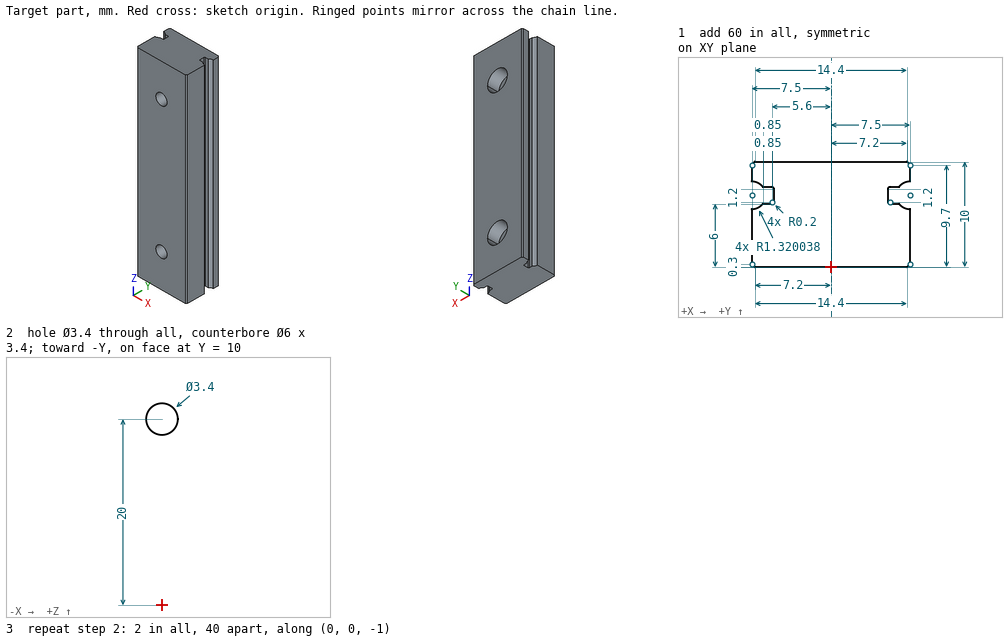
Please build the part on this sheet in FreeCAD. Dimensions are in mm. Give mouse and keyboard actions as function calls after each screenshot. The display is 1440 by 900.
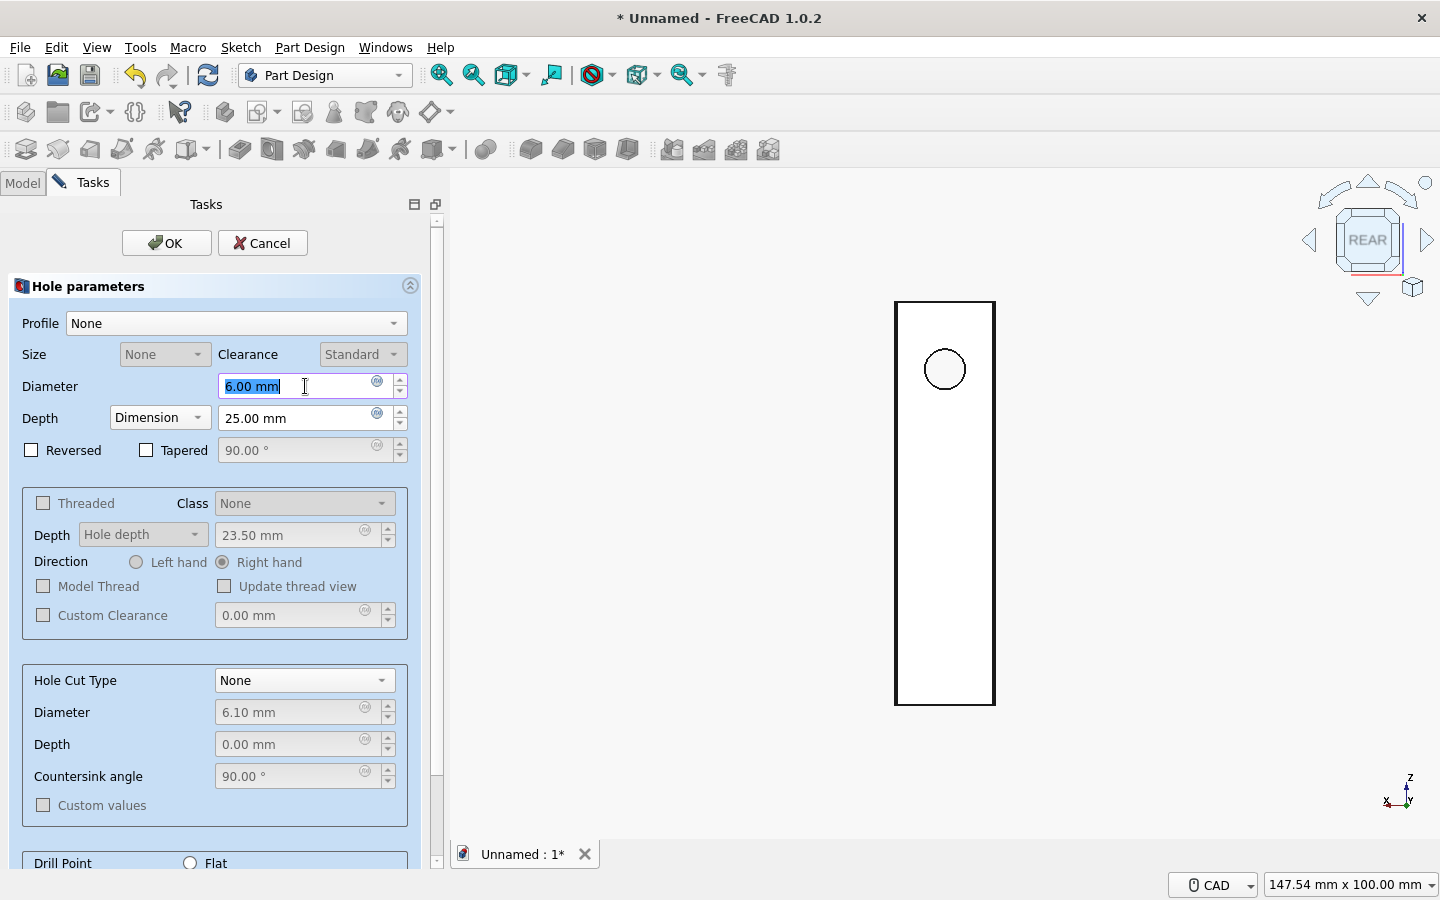
text(3.4)
key(Tab)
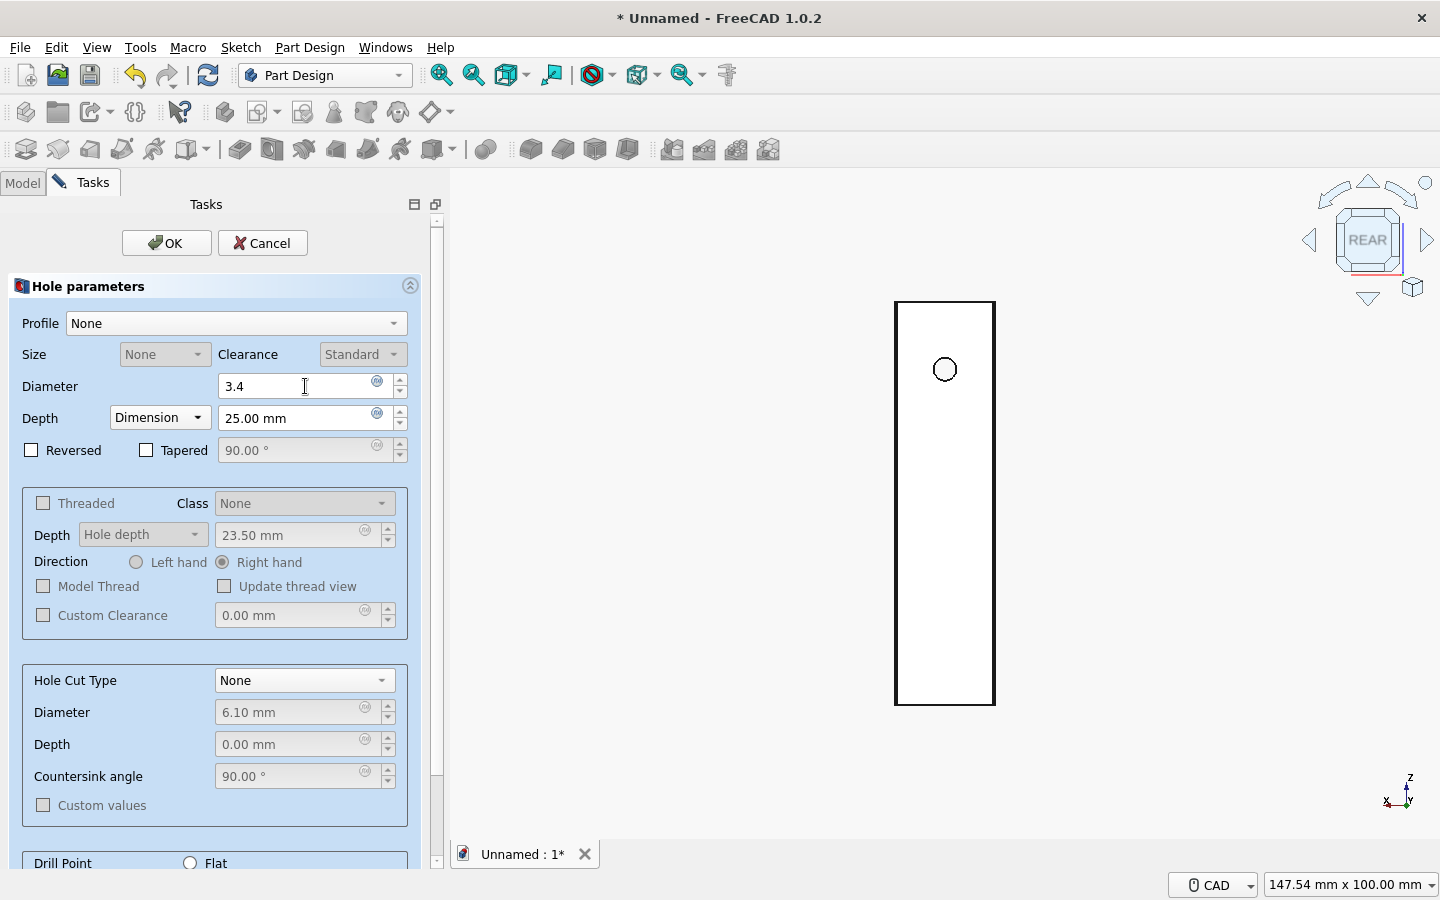
click(161, 418)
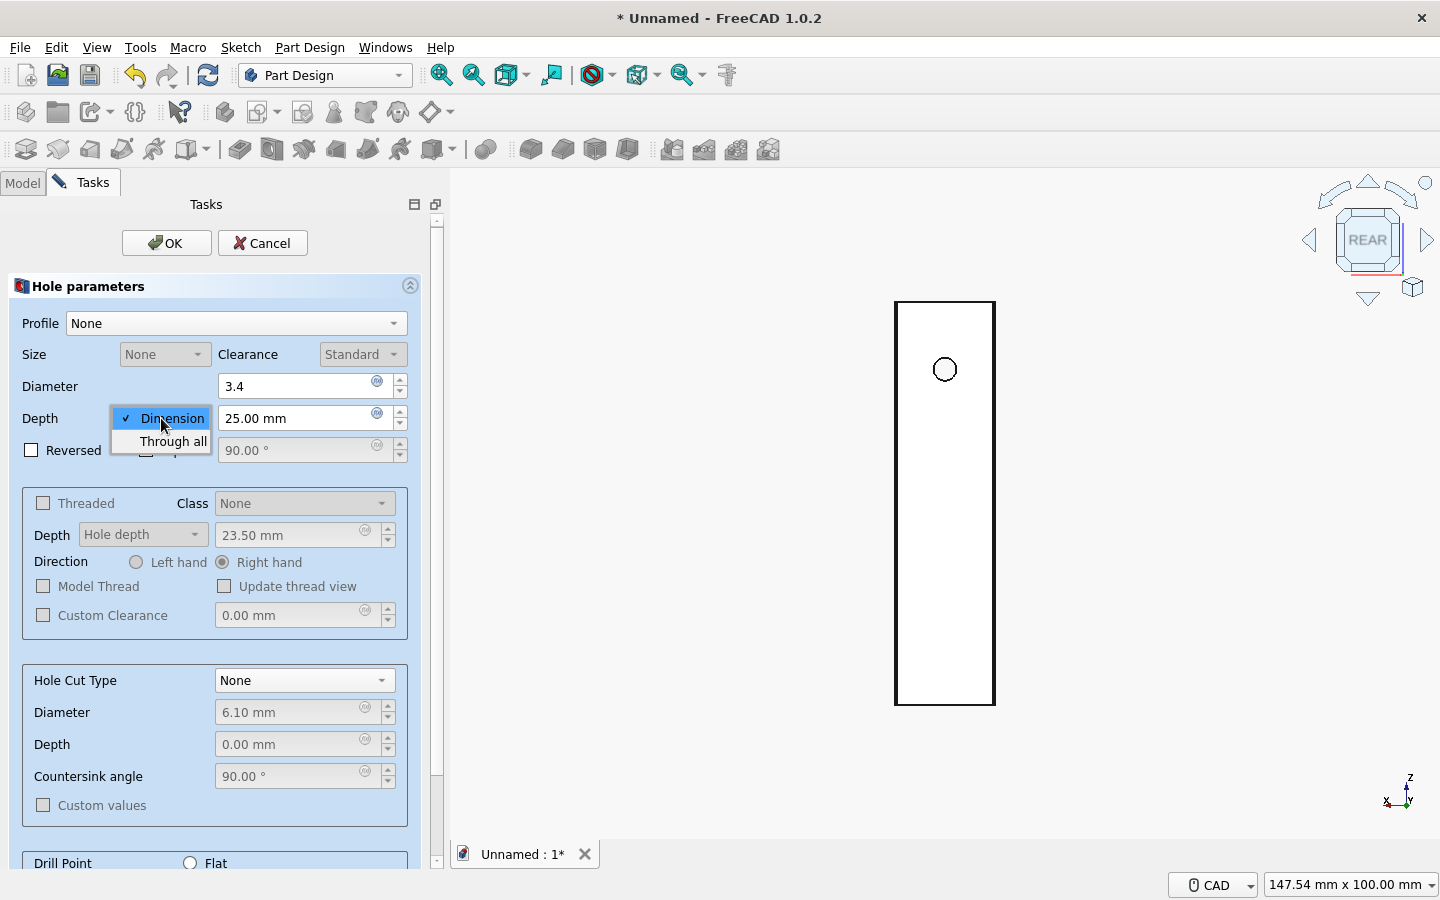
click(160, 442)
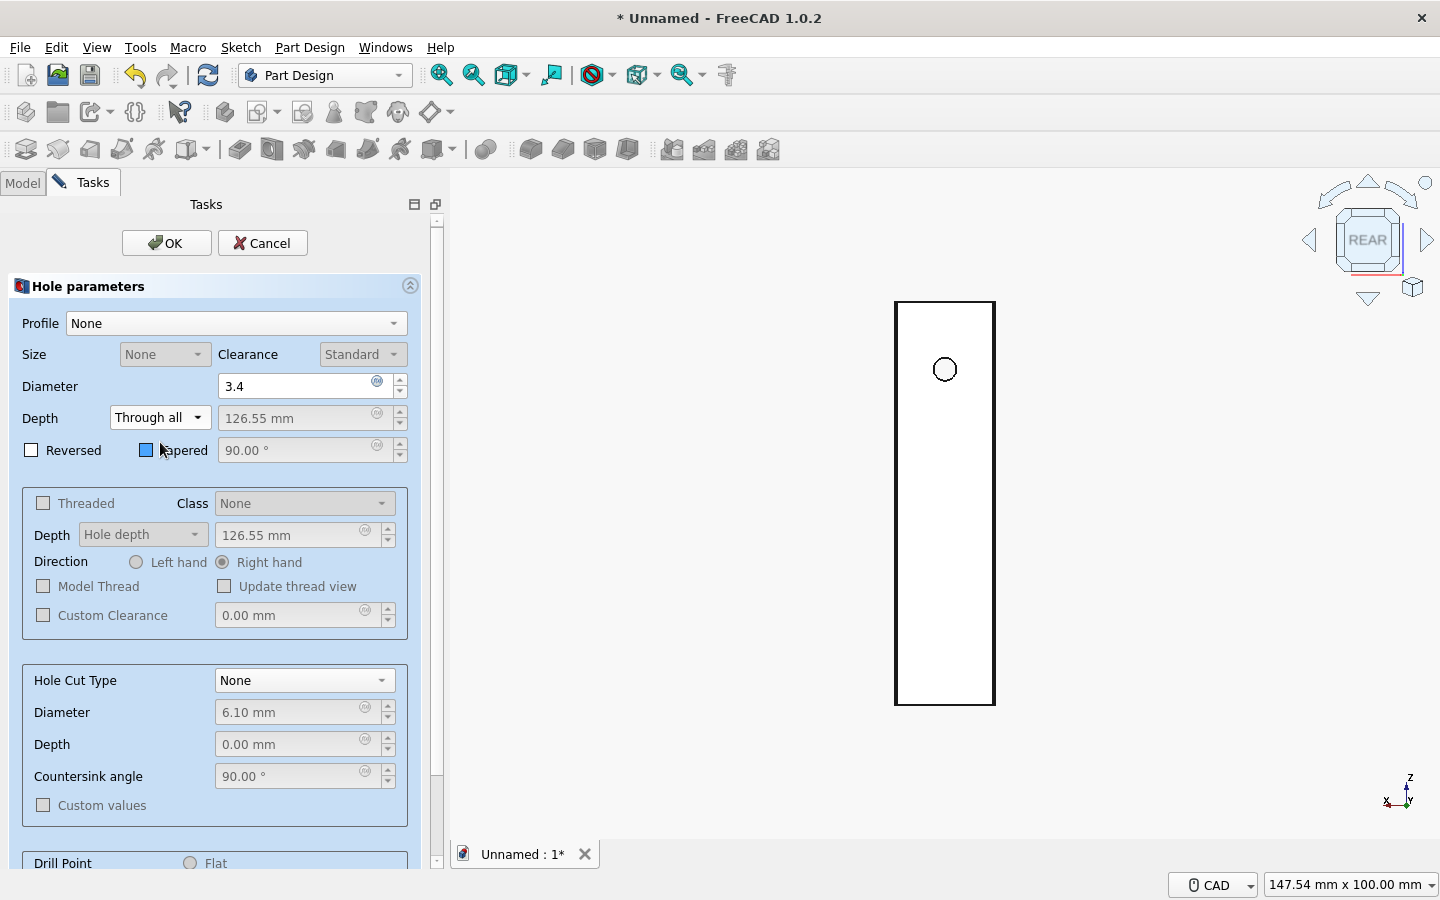
click(306, 680)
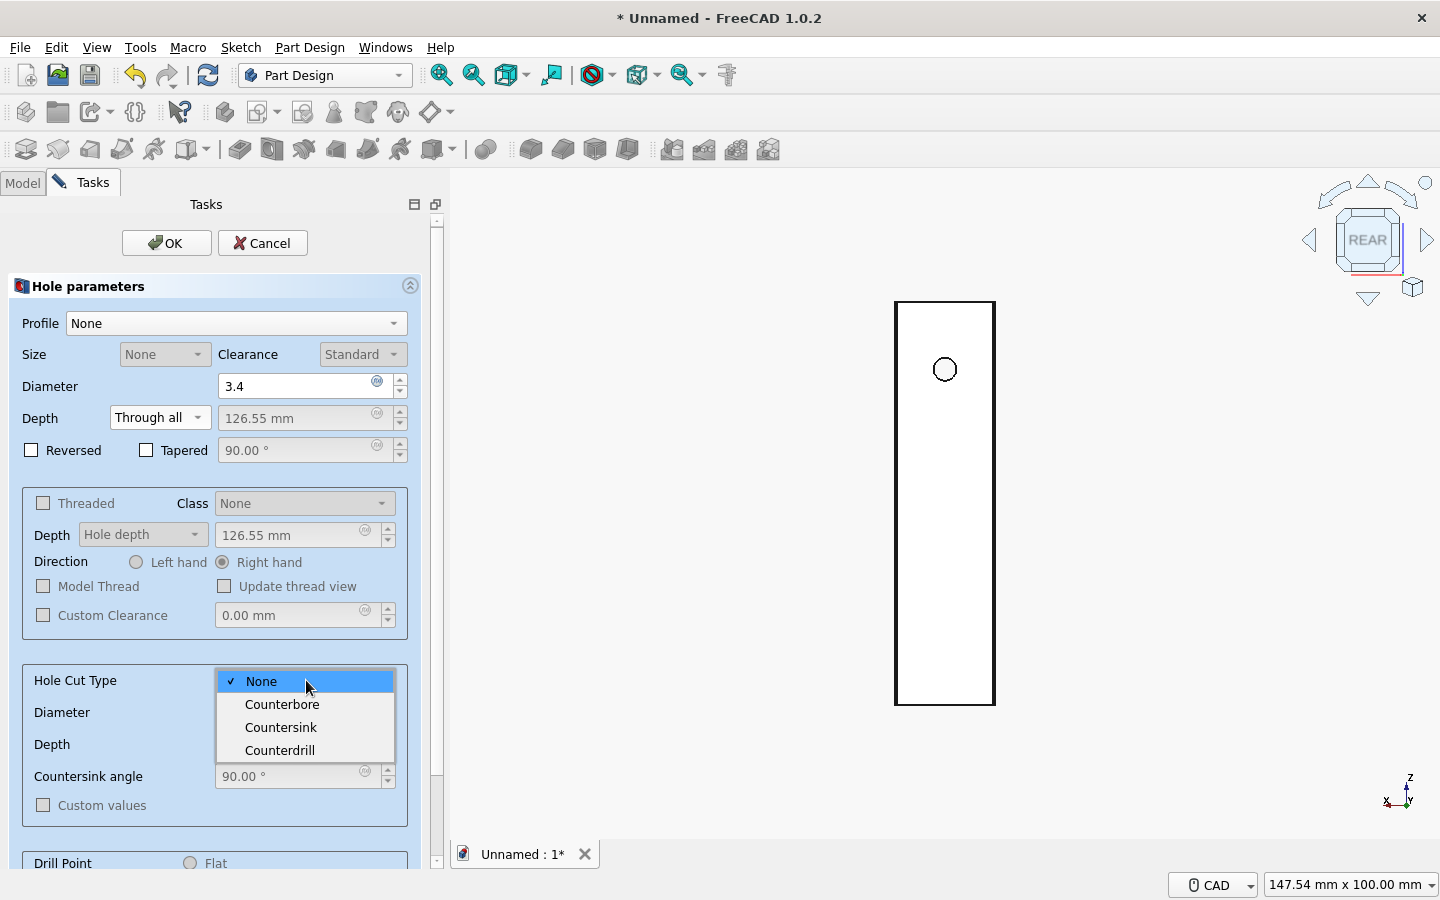
click(304, 704)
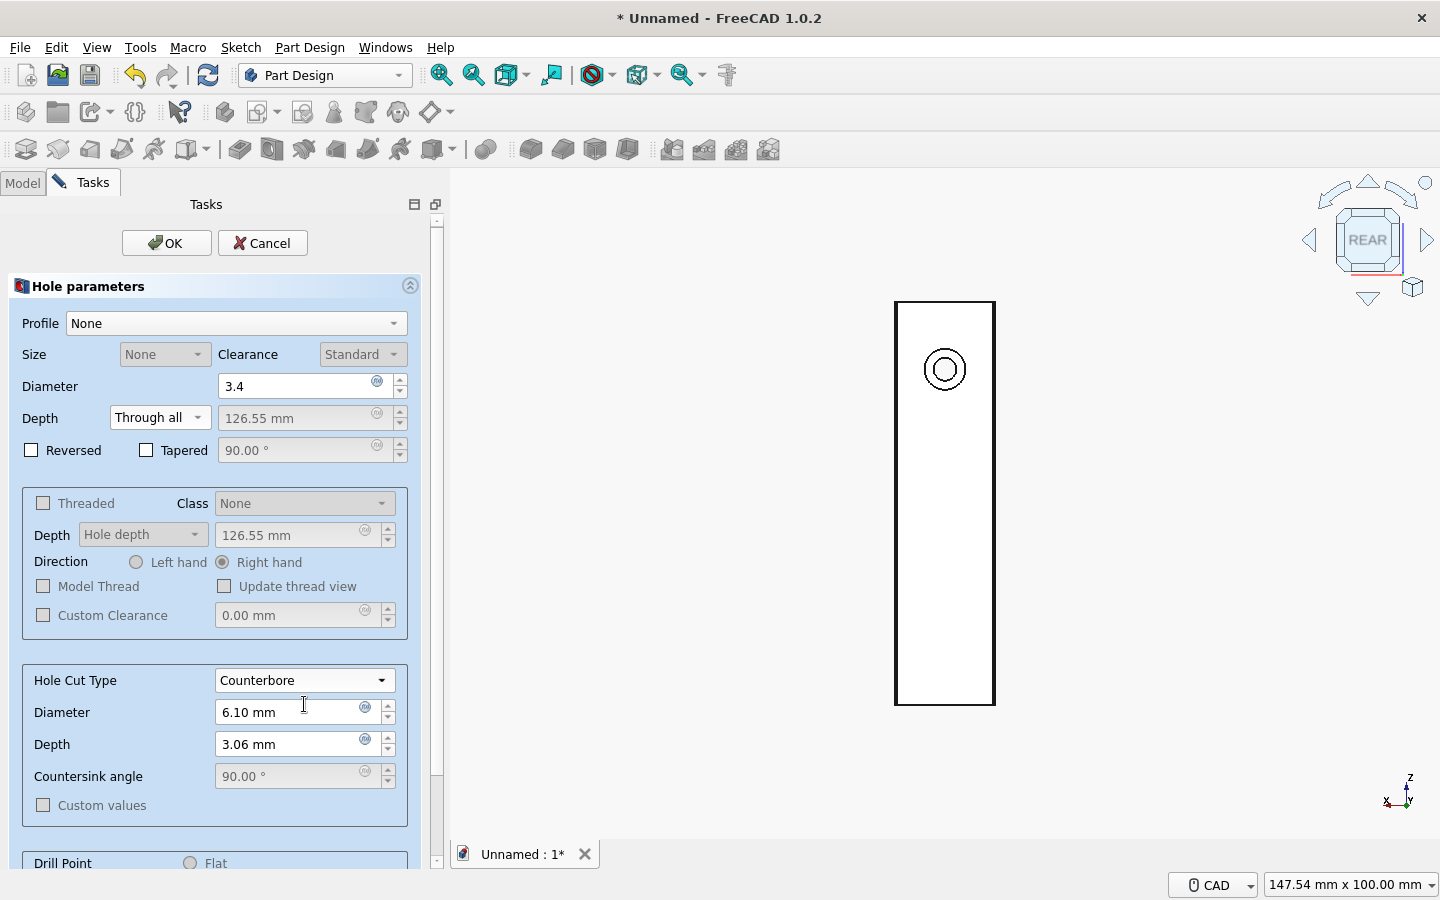
triple_click(298, 712)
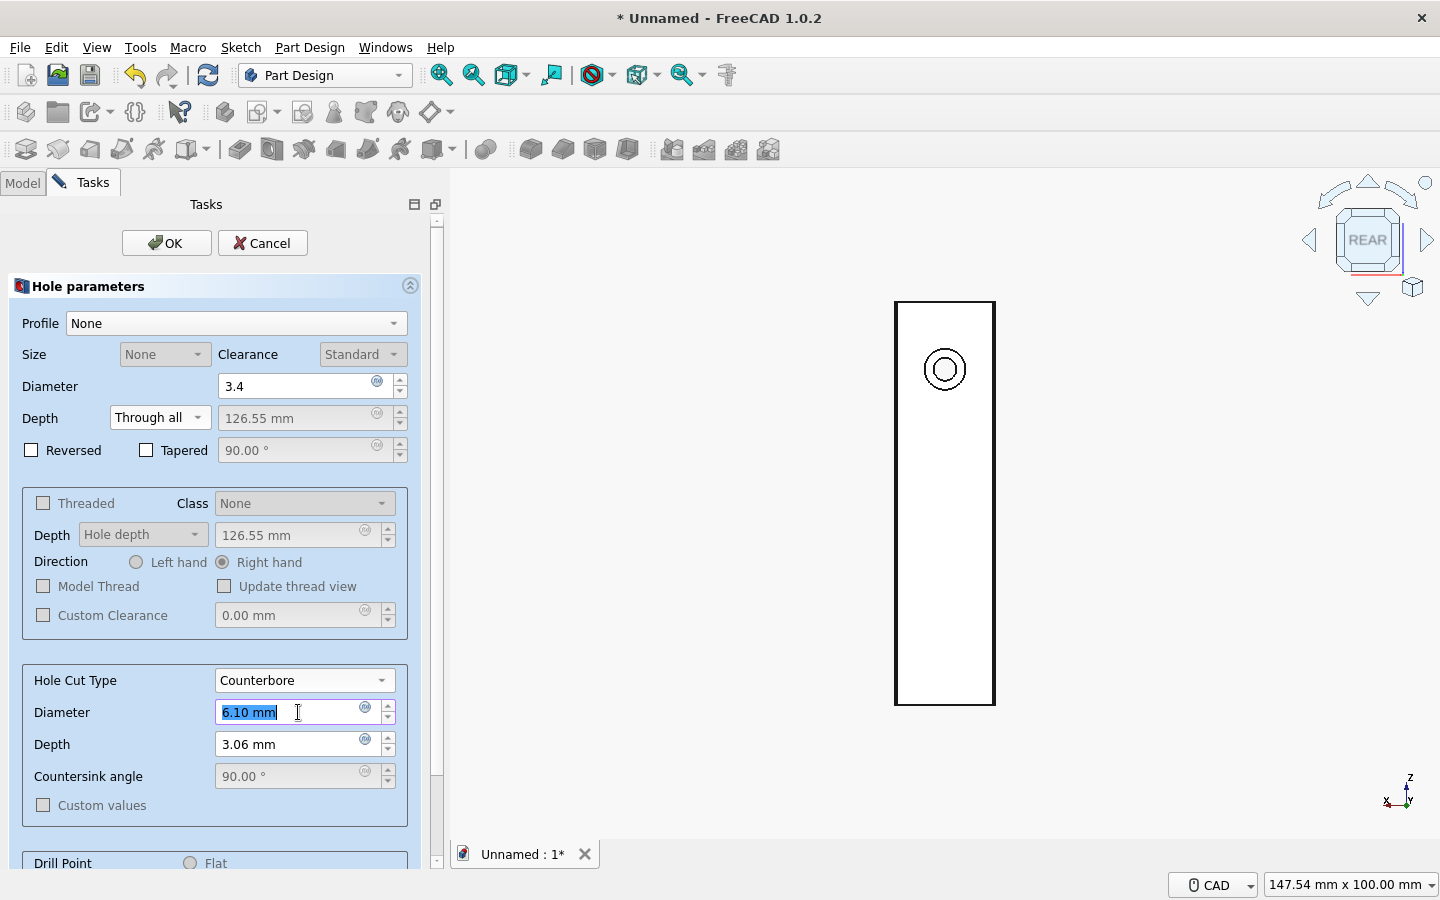
text(6)
key(Tab)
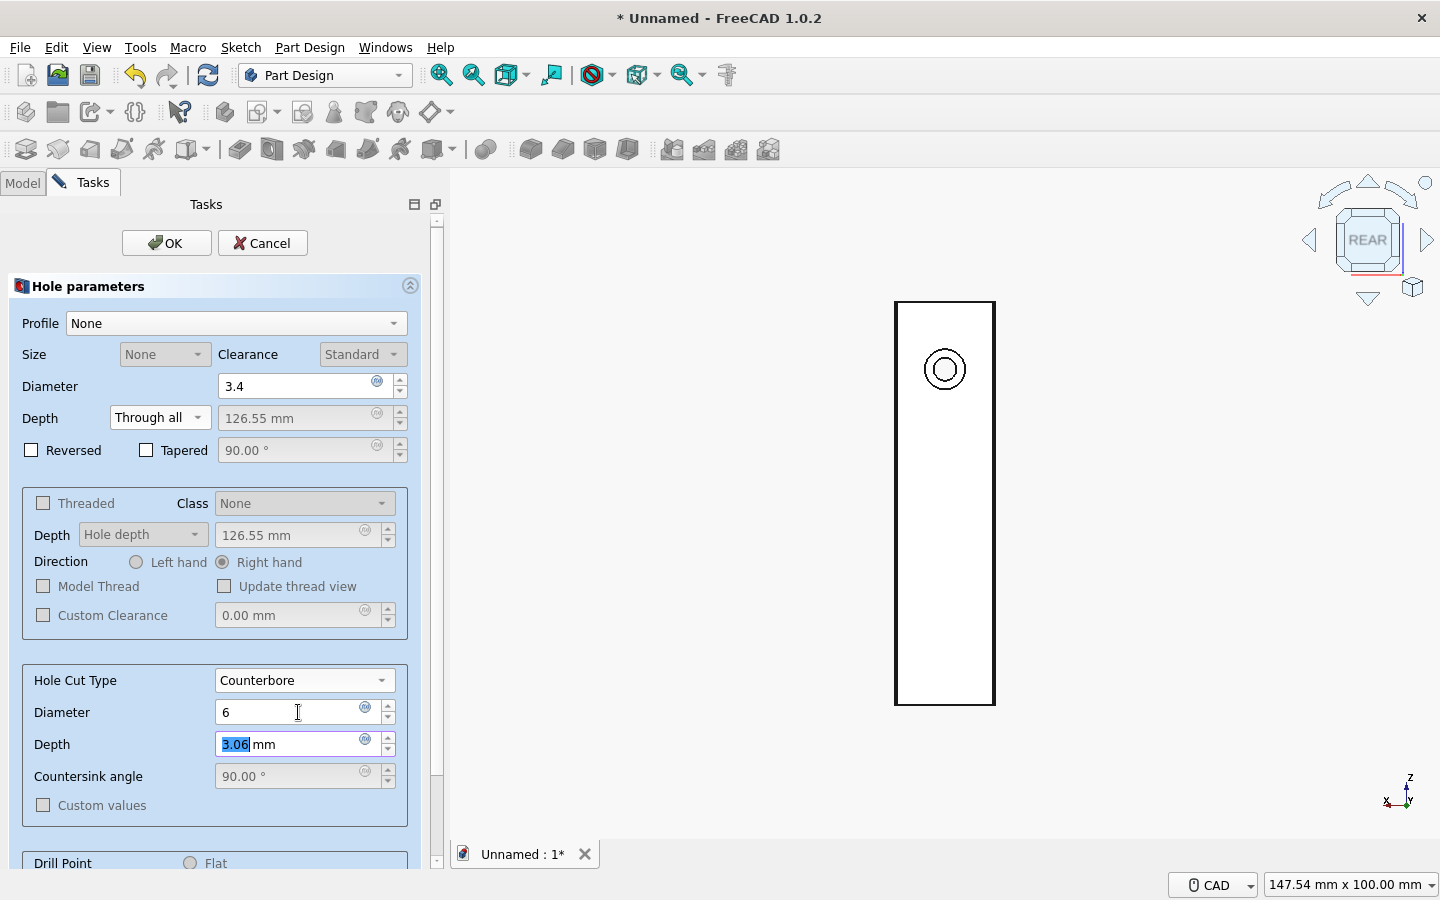
text(3.4)
key(Tab)